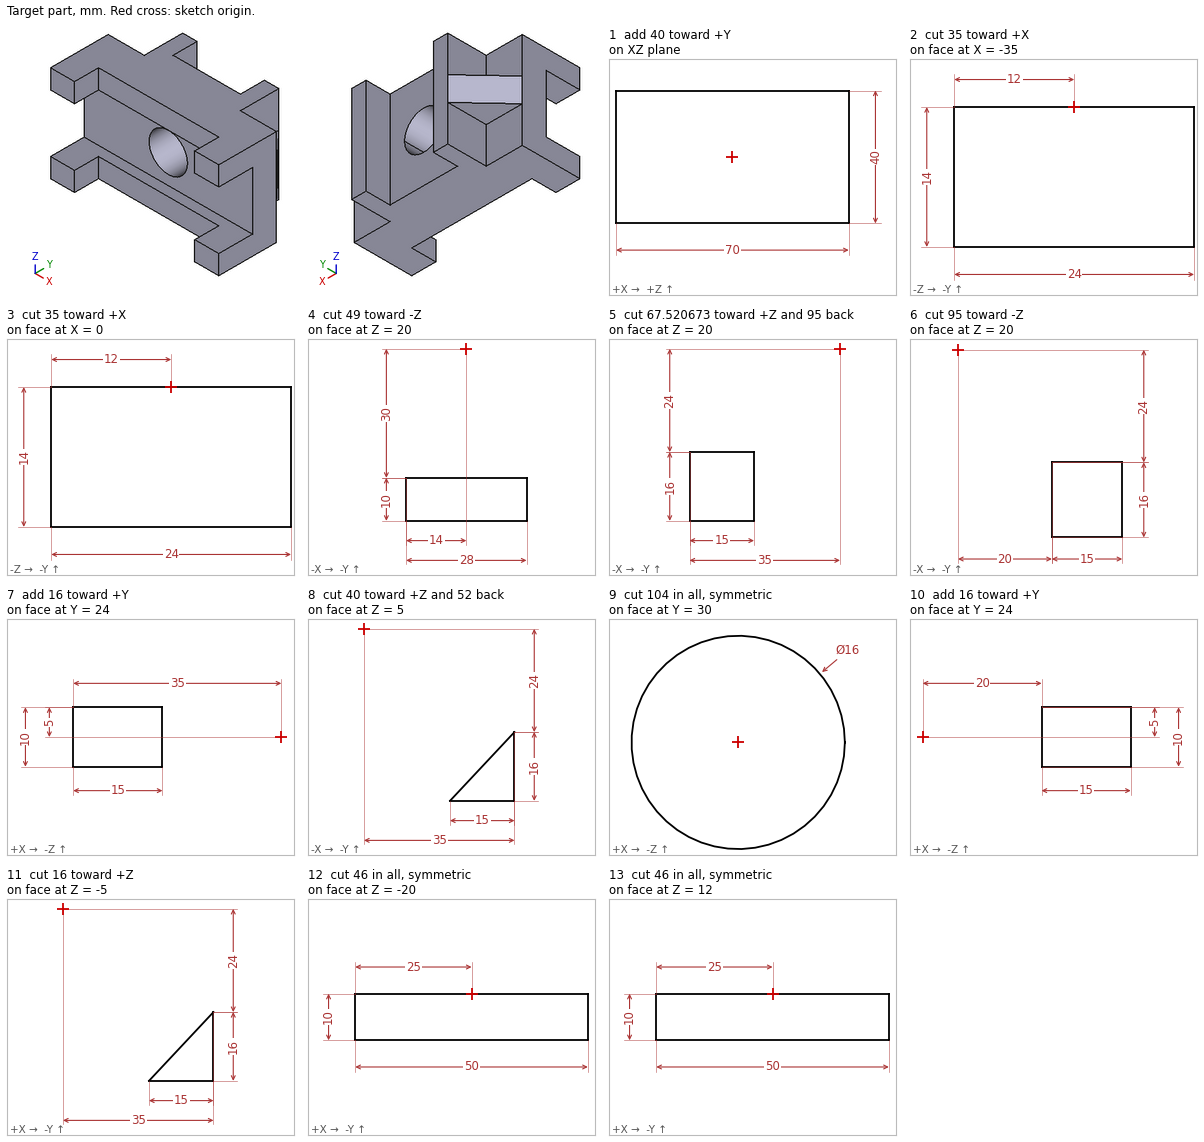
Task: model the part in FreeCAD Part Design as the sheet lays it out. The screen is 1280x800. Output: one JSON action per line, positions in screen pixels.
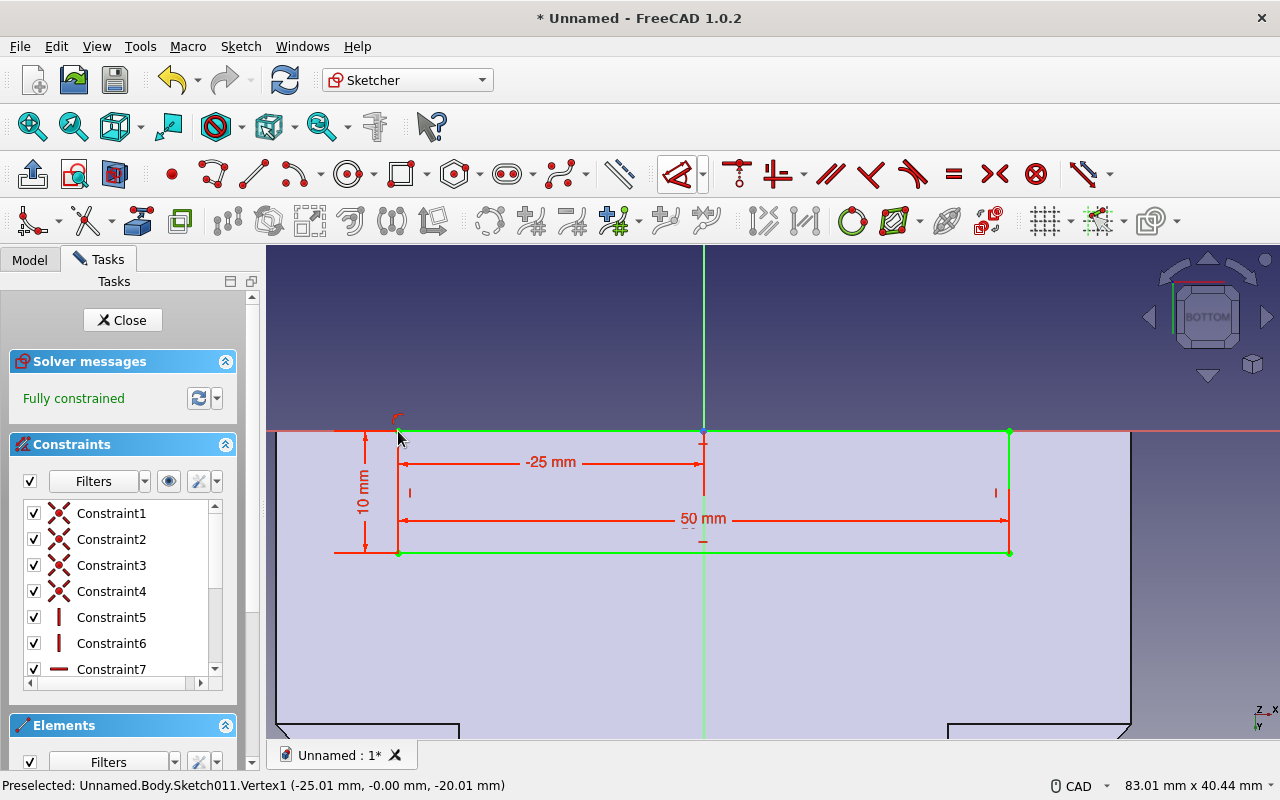
{"action": "left_click", "coordinate": [123, 320]}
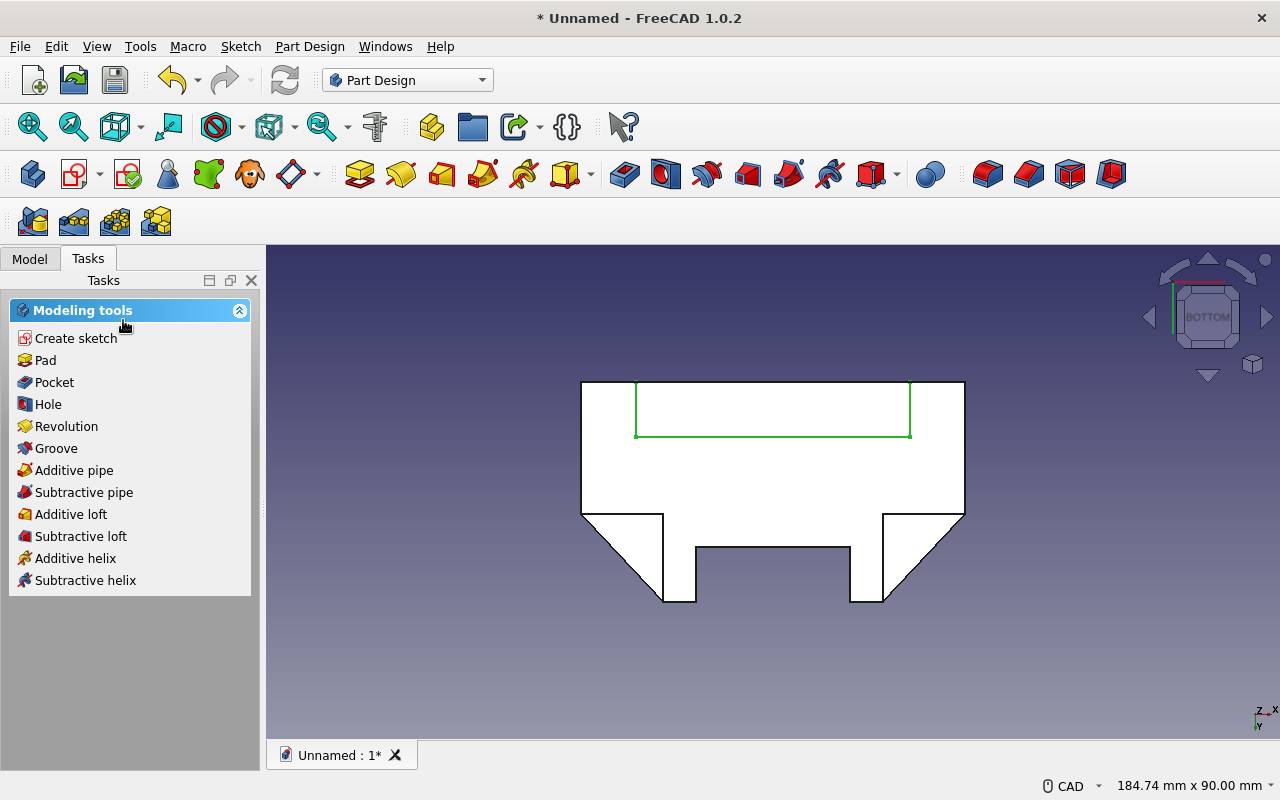
{"action": "left_click", "coordinate": [625, 174]}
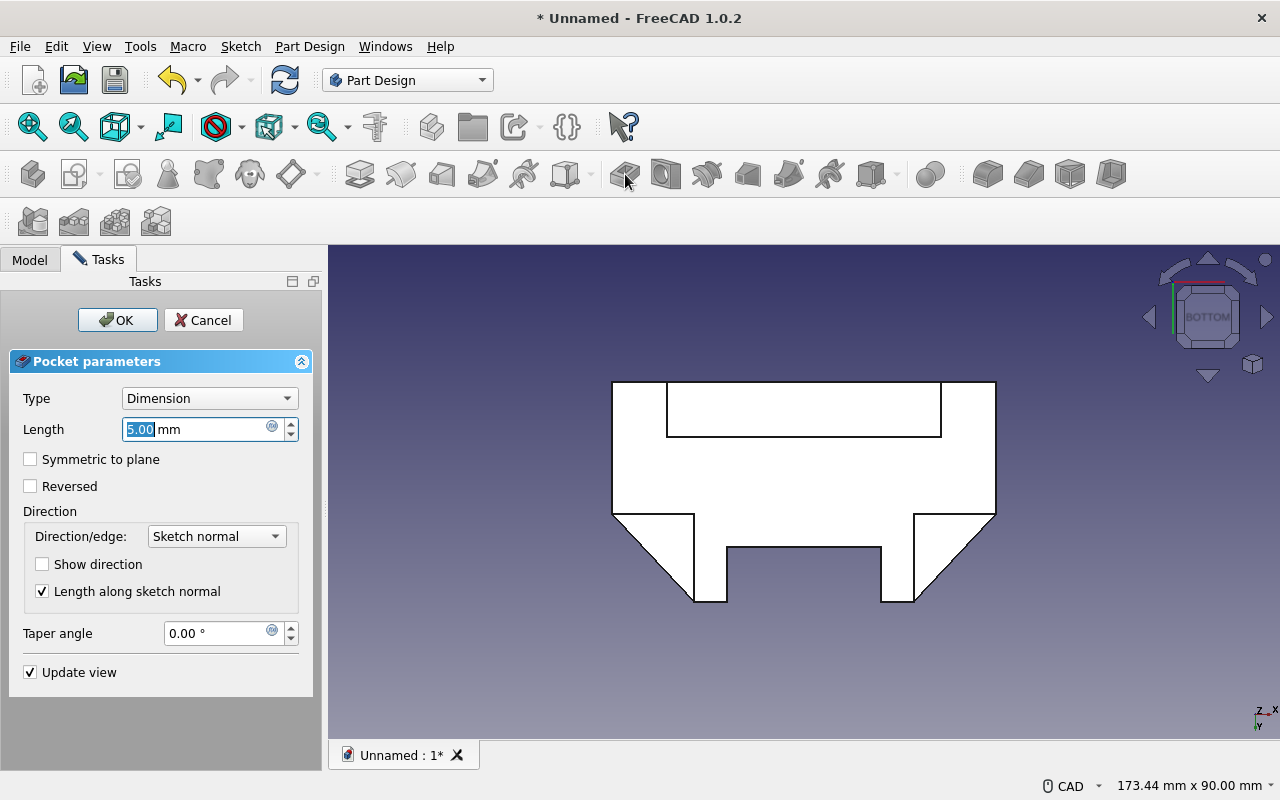
{"action": "type", "text": "46"}
{"action": "key", "text": "Tab"}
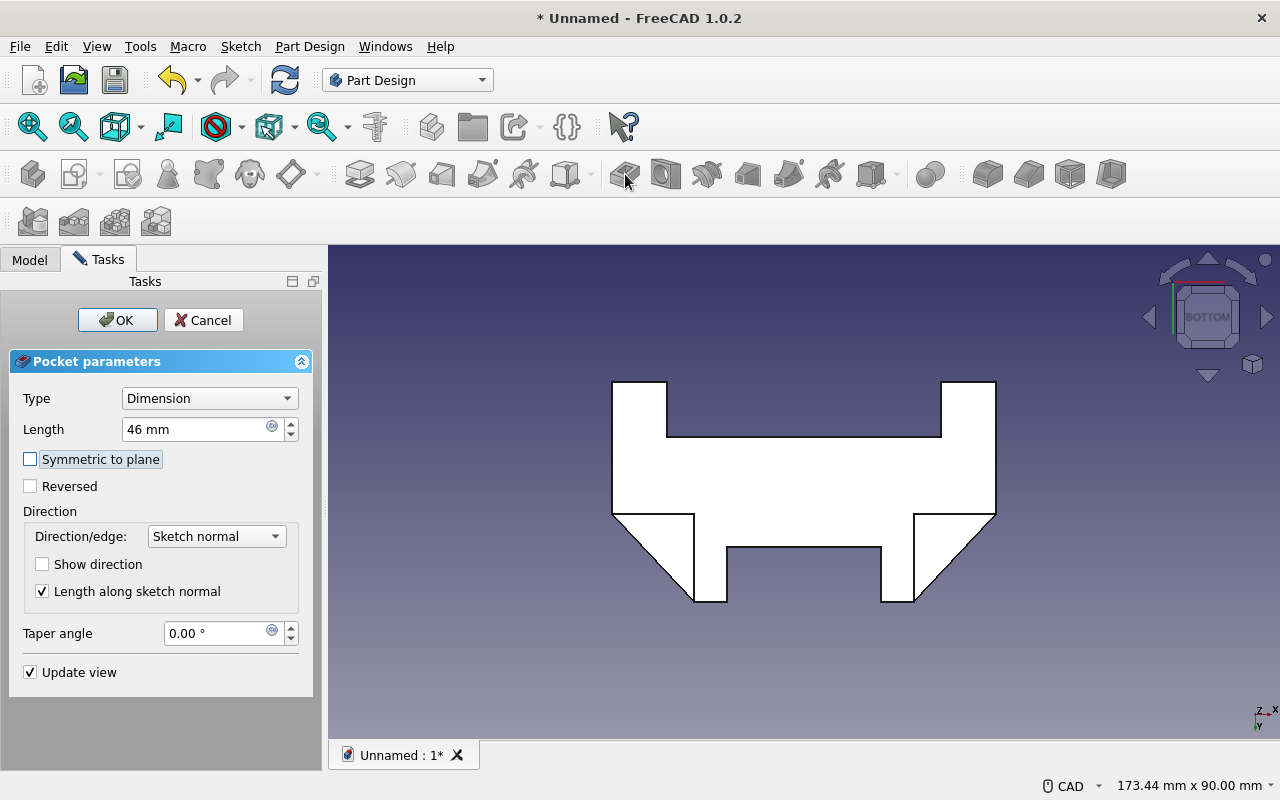
{"action": "left_click", "coordinate": [31, 459]}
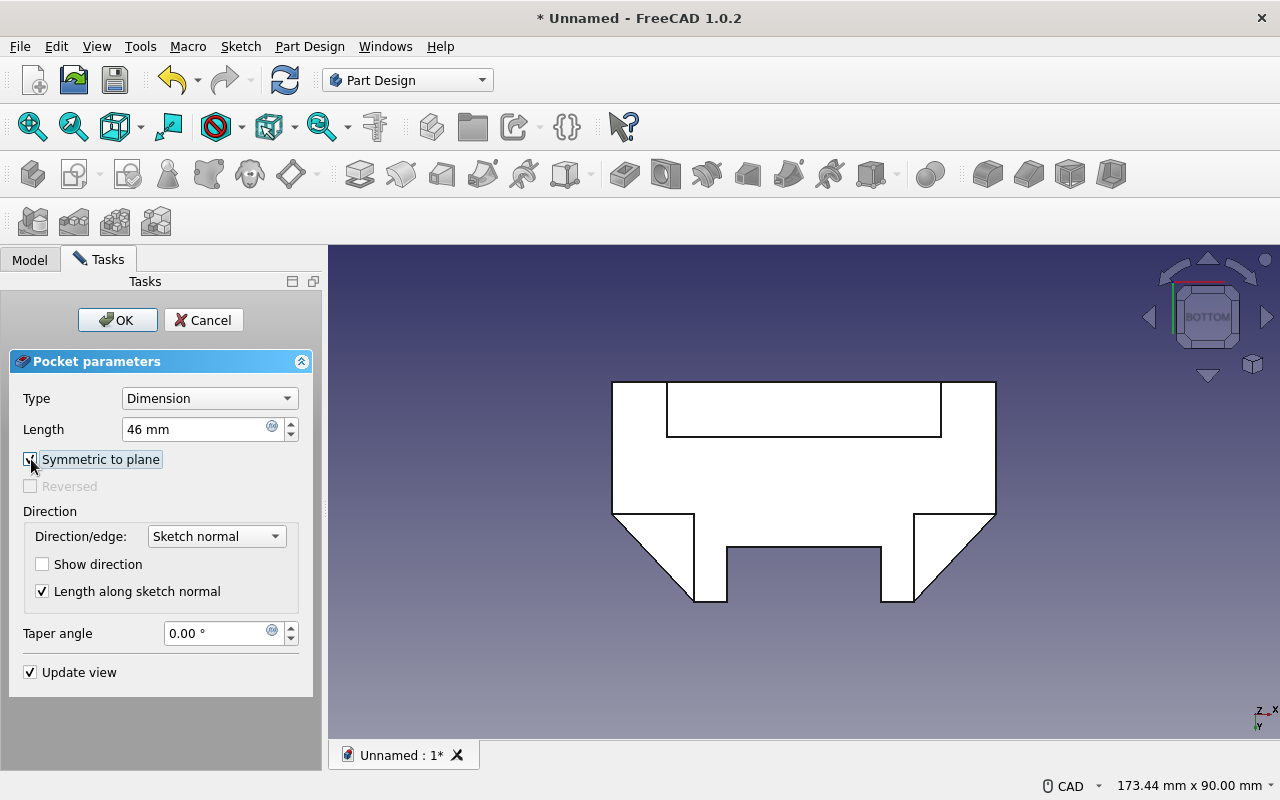
{"action": "left_click", "coordinate": [118, 320]}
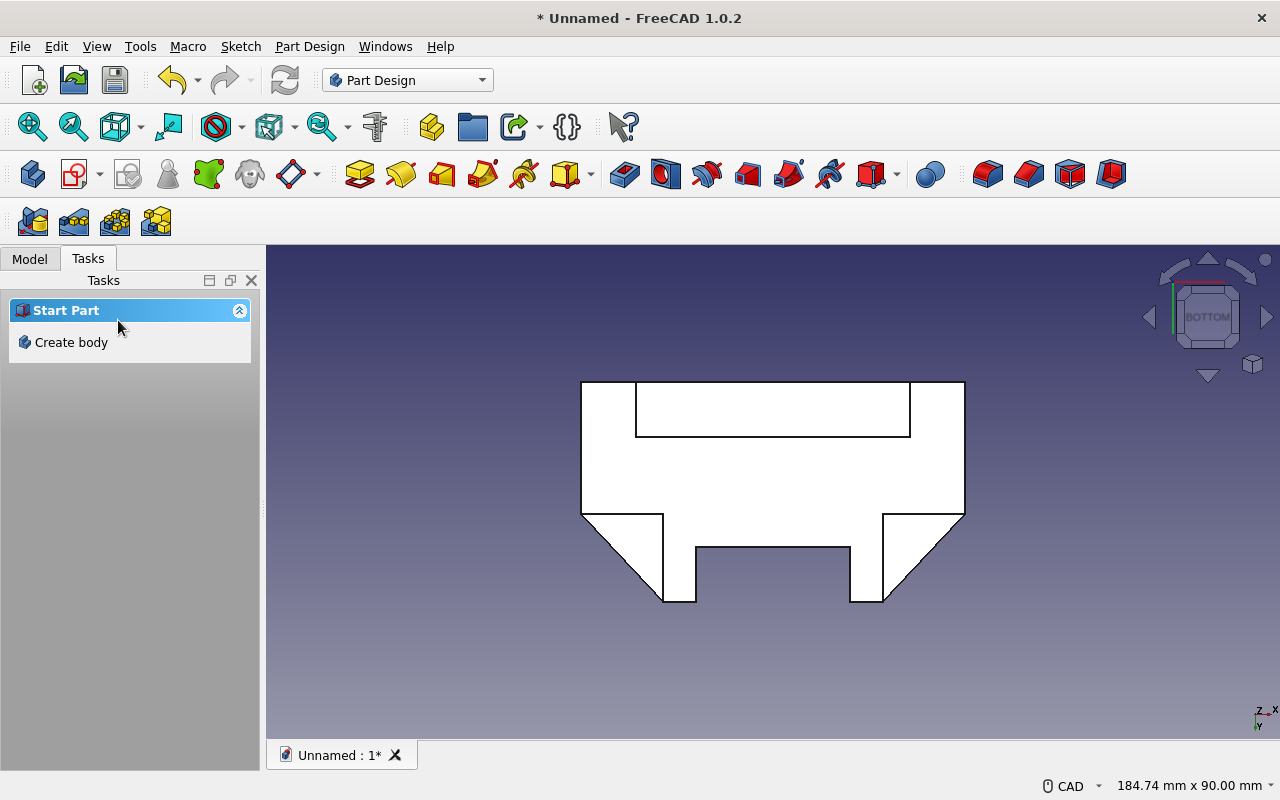
{"action": "key", "text": "v f"}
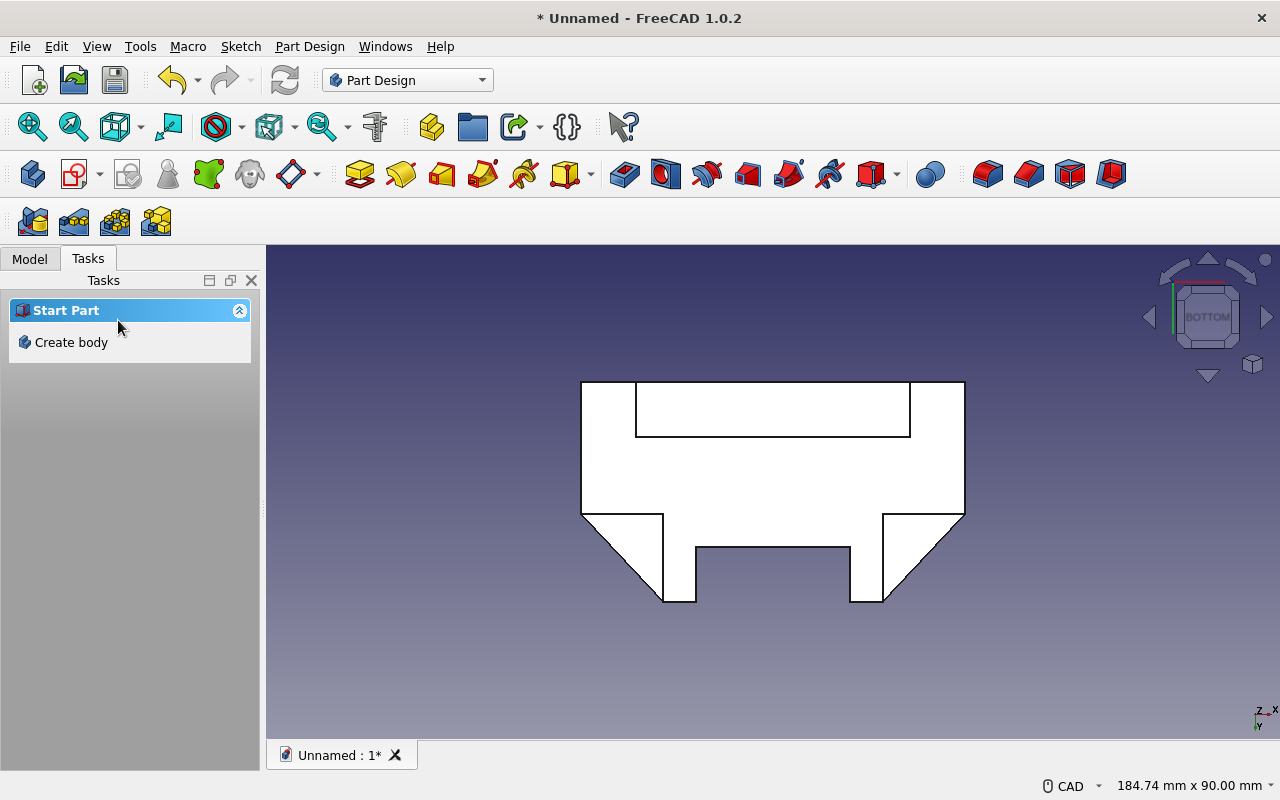
{"action": "left_click", "coordinate": [883, 420]}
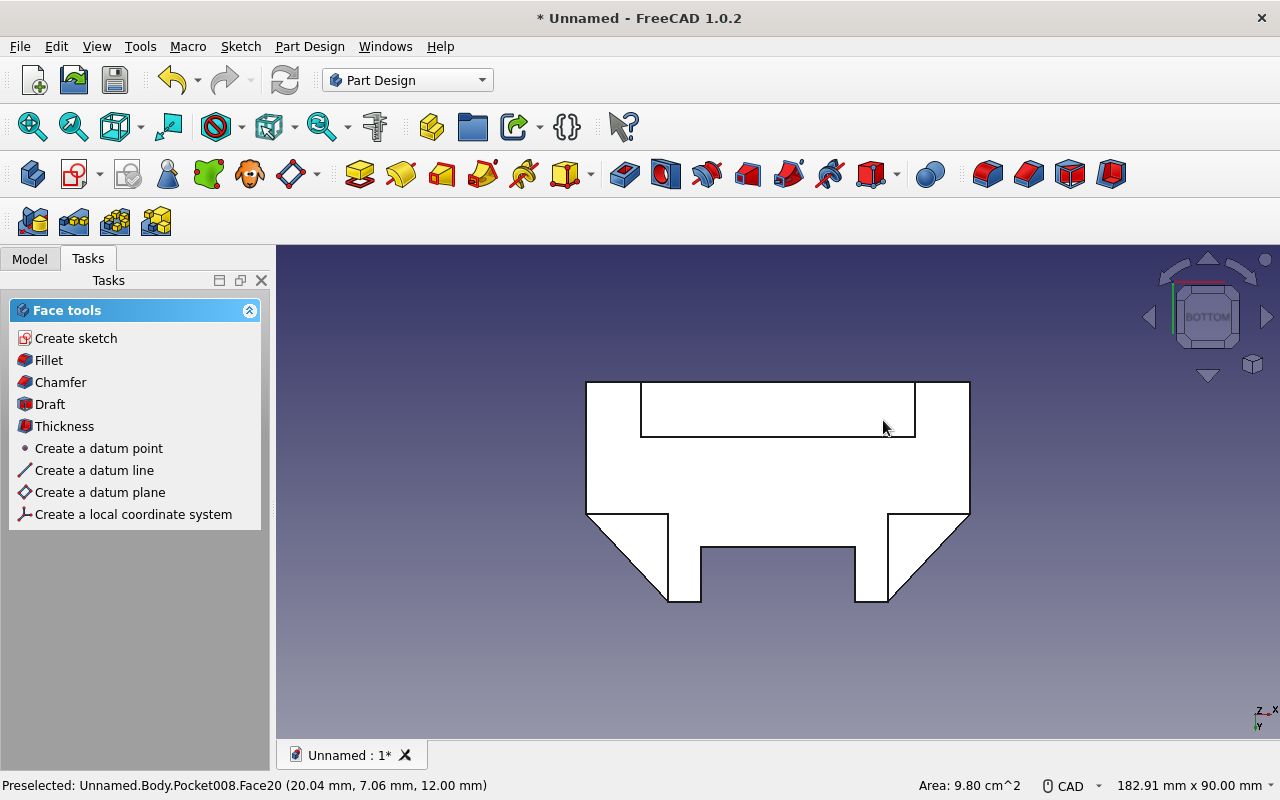
{"action": "left_click", "coordinate": [74, 174]}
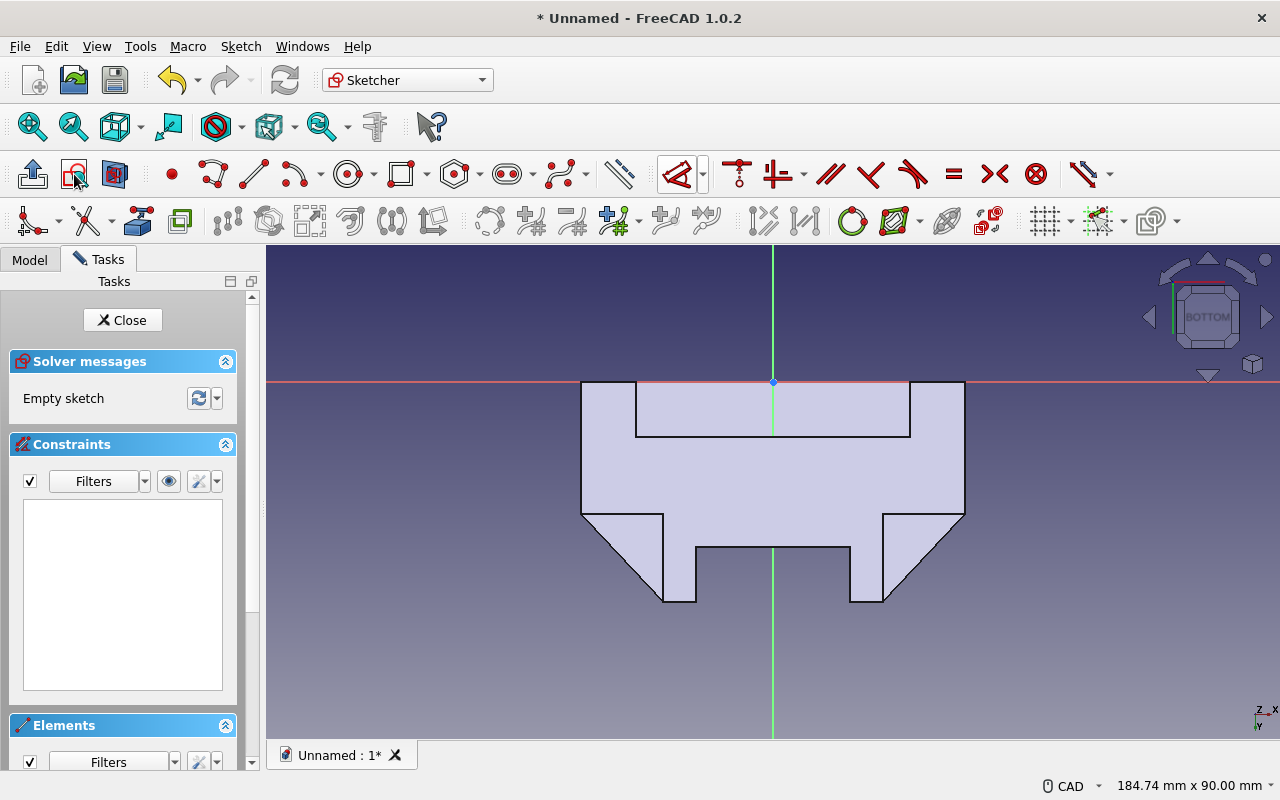
{"action": "scroll", "coordinate": [829, 342], "scroll_direction": "up", "scroll_amount": 4}